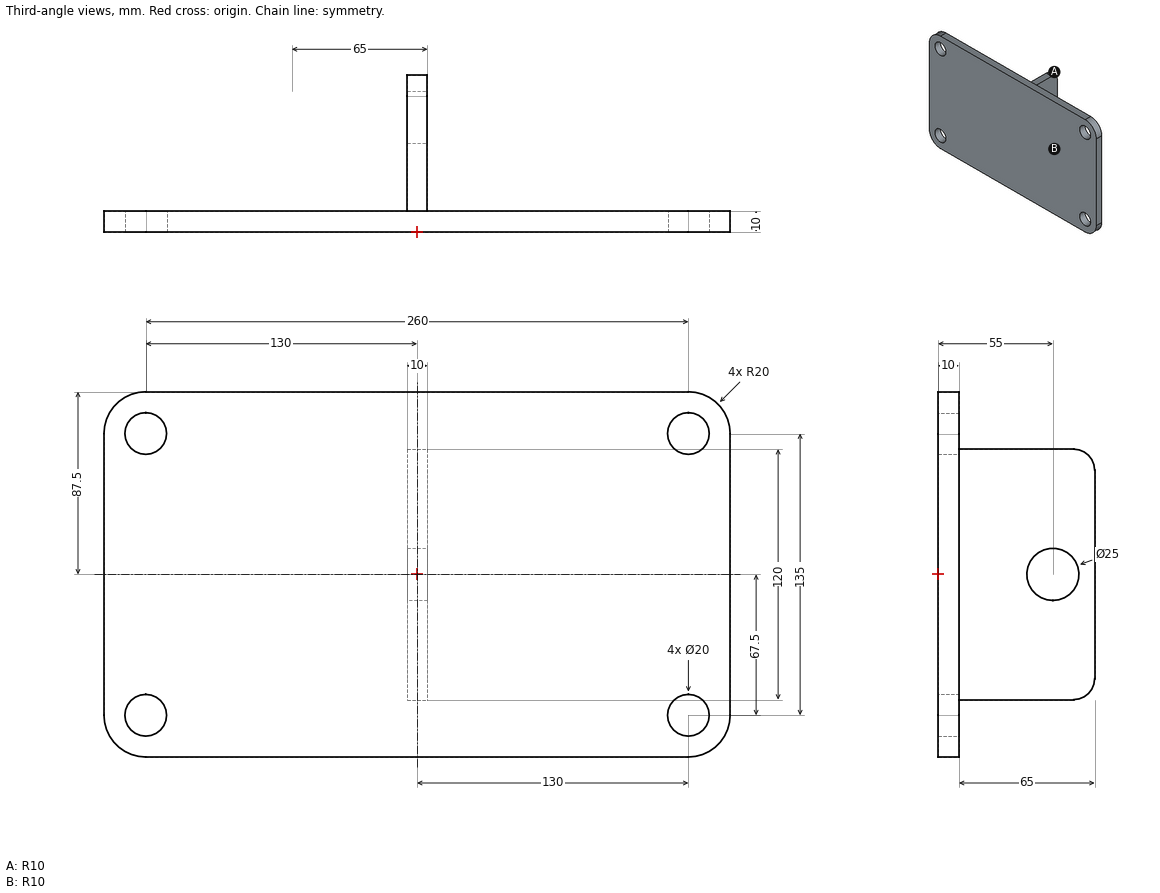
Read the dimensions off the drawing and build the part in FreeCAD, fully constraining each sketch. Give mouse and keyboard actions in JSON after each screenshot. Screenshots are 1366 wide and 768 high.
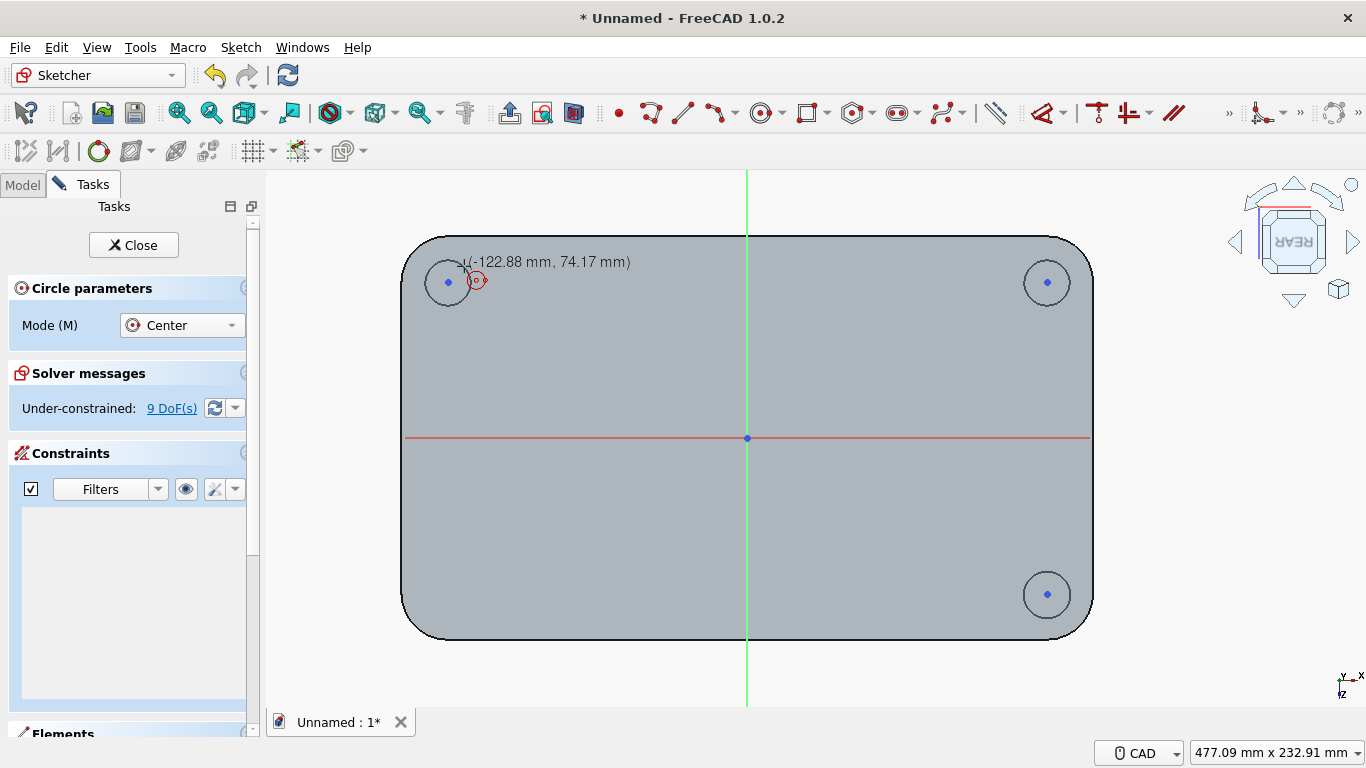
{"action": "left_click", "coordinate": [448, 594]}
{"action": "left_click", "coordinate": [464, 577]}
{"action": "key", "text": "Escape"}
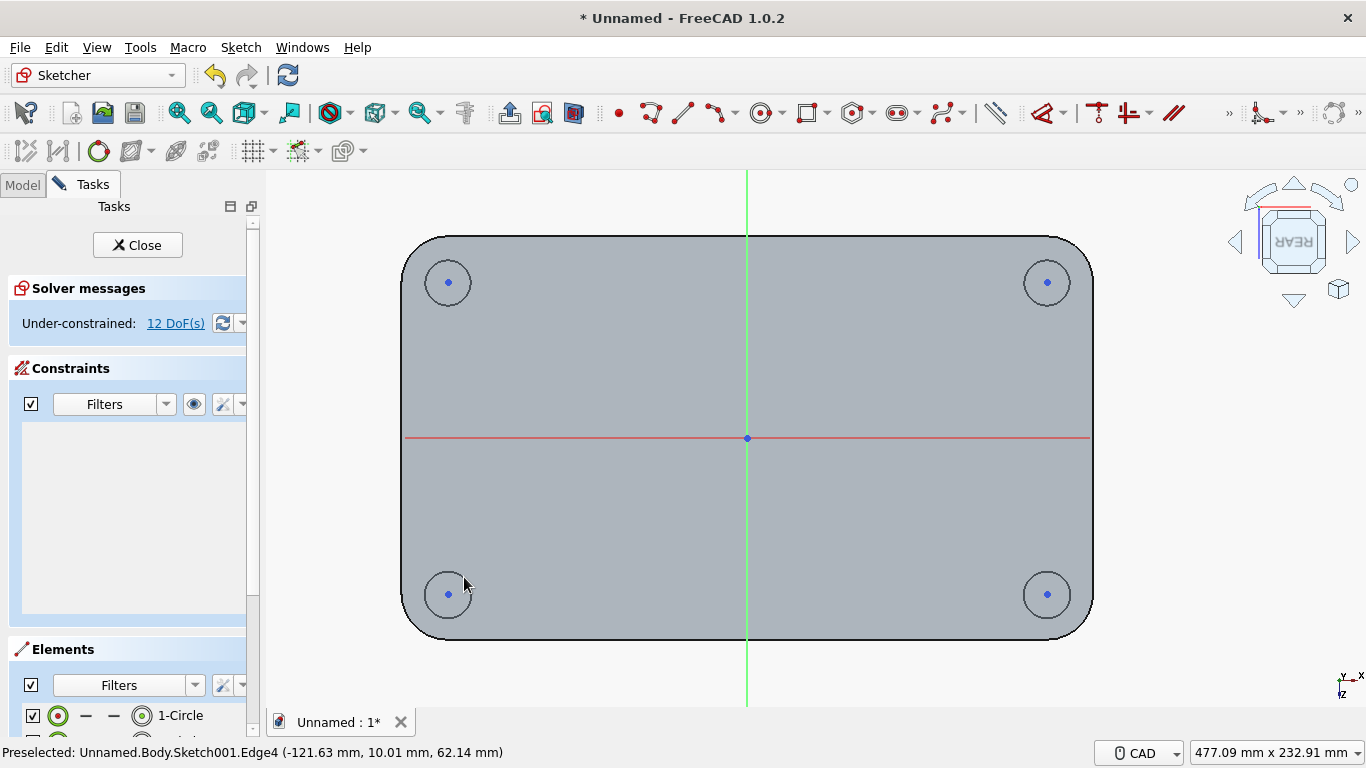
{"action": "left_click", "coordinate": [1063, 267]}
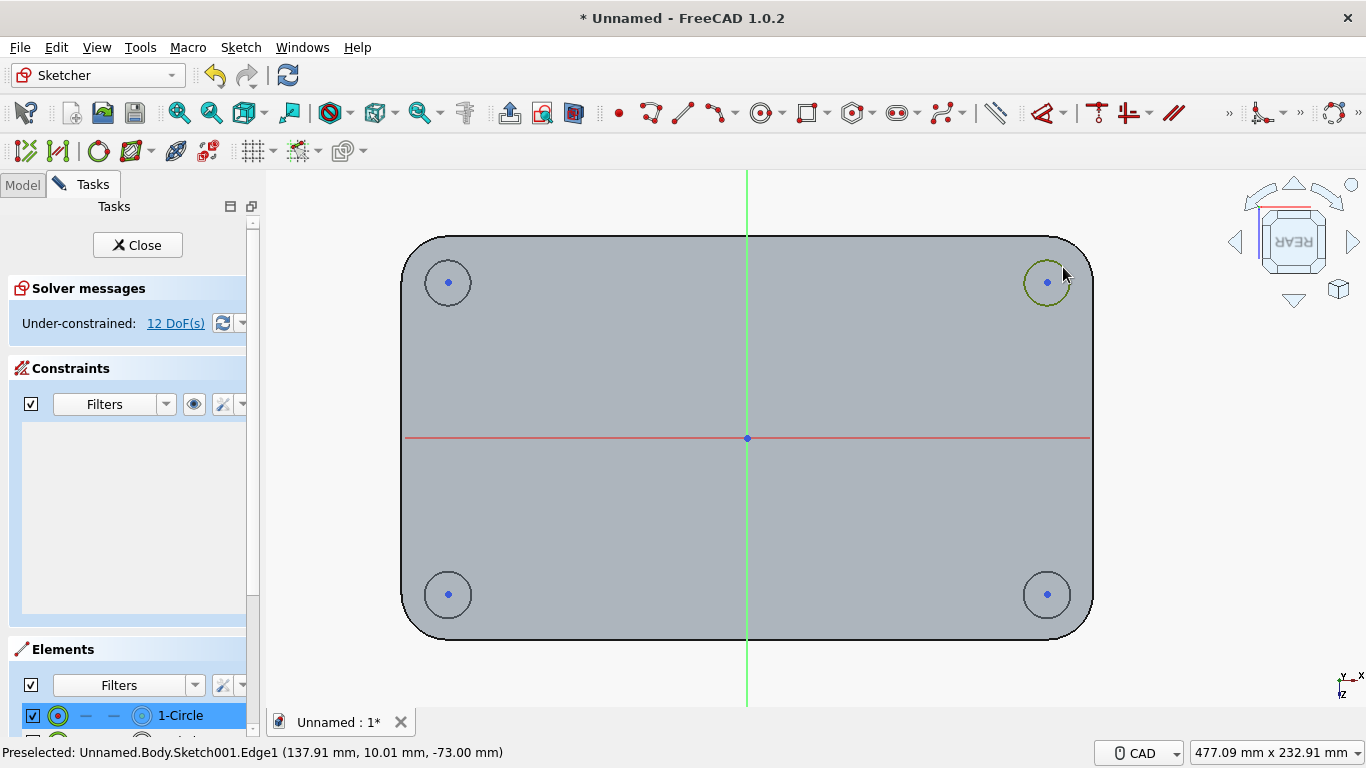
{"action": "left_click", "coordinate": [1063, 578]}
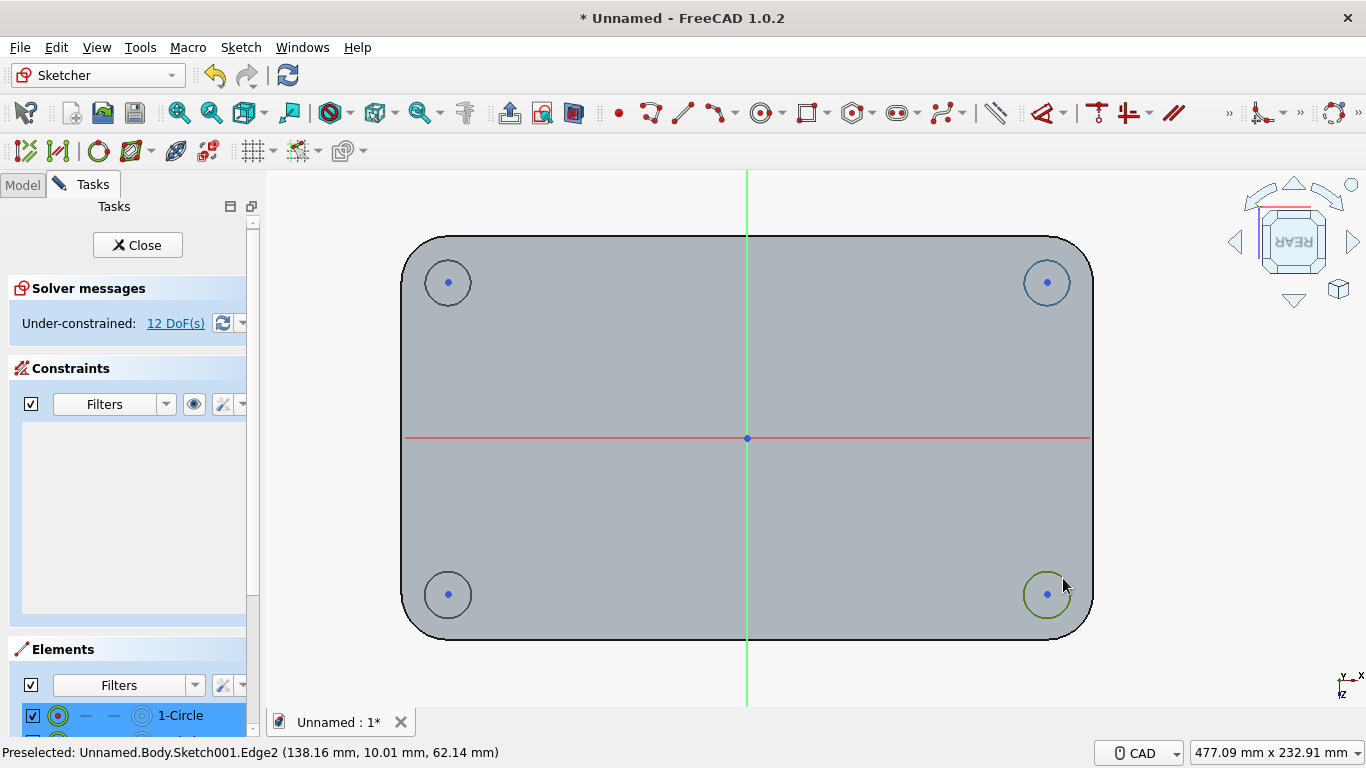
{"action": "left_click", "coordinate": [464, 267]}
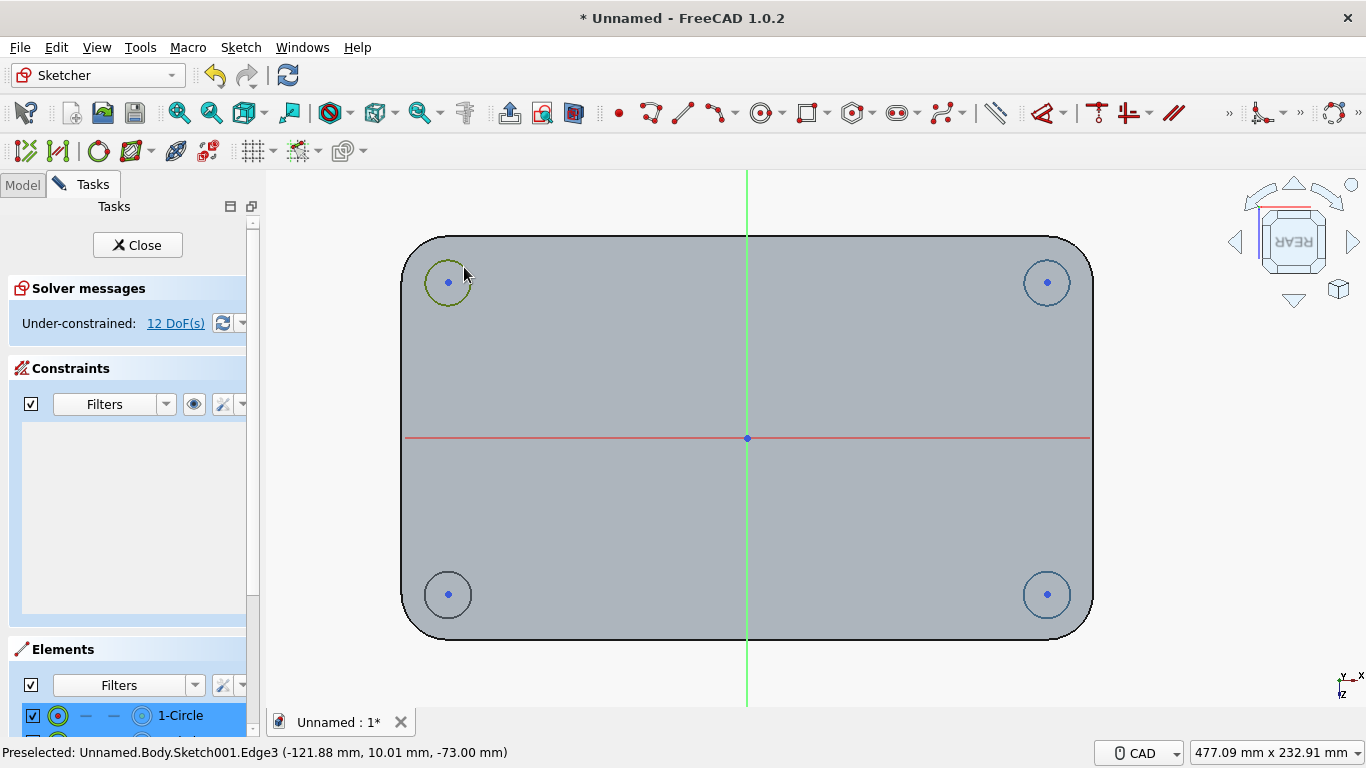
{"action": "left_click", "coordinate": [464, 578]}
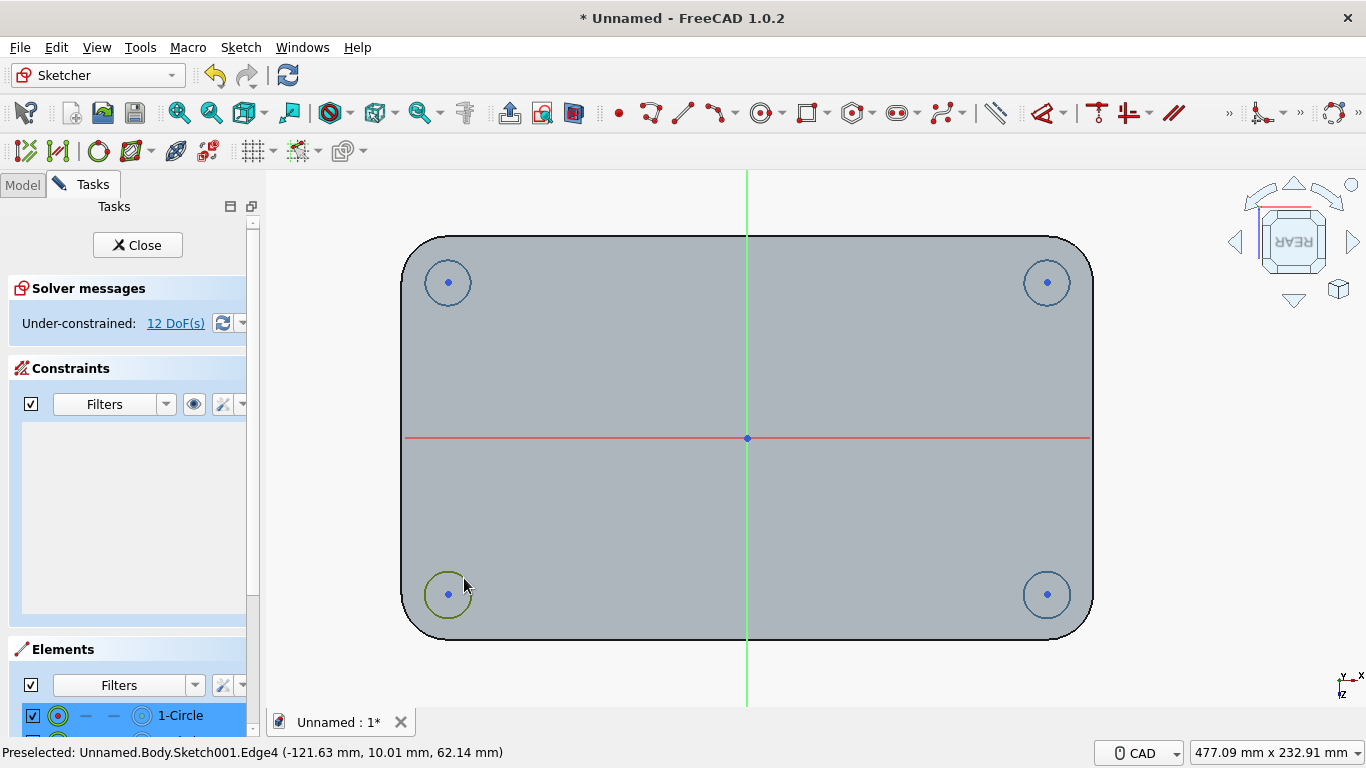
{"action": "key", "text": "e"}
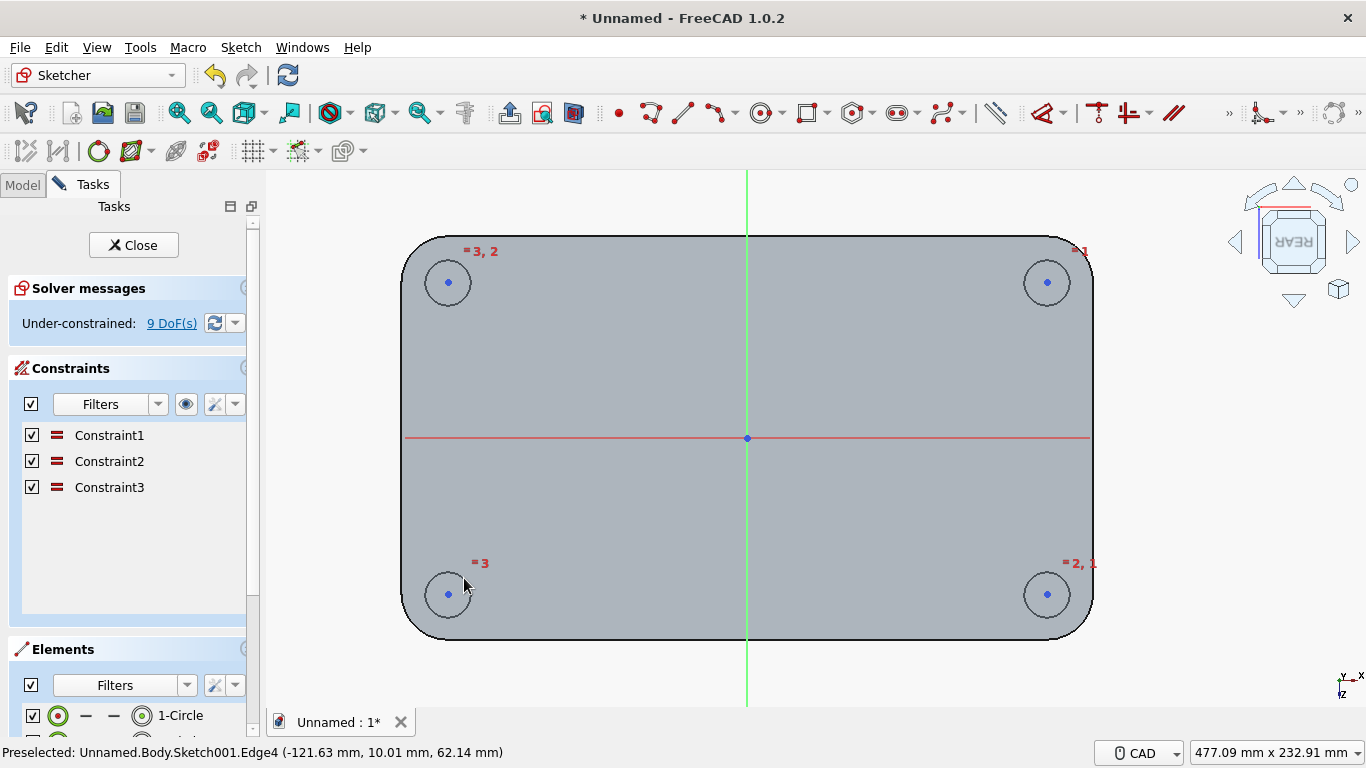
{"action": "left_click", "coordinate": [1047, 283]}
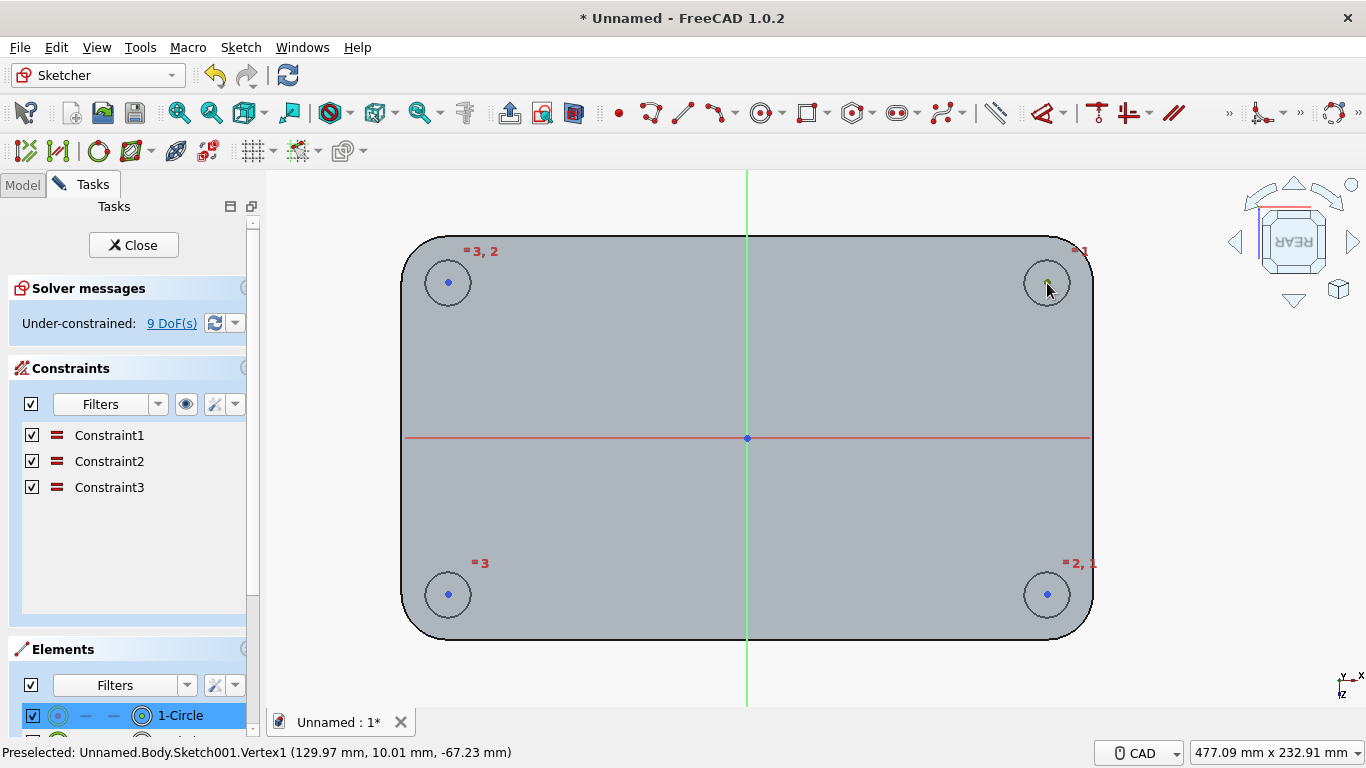
{"action": "left_click", "coordinate": [1047, 595]}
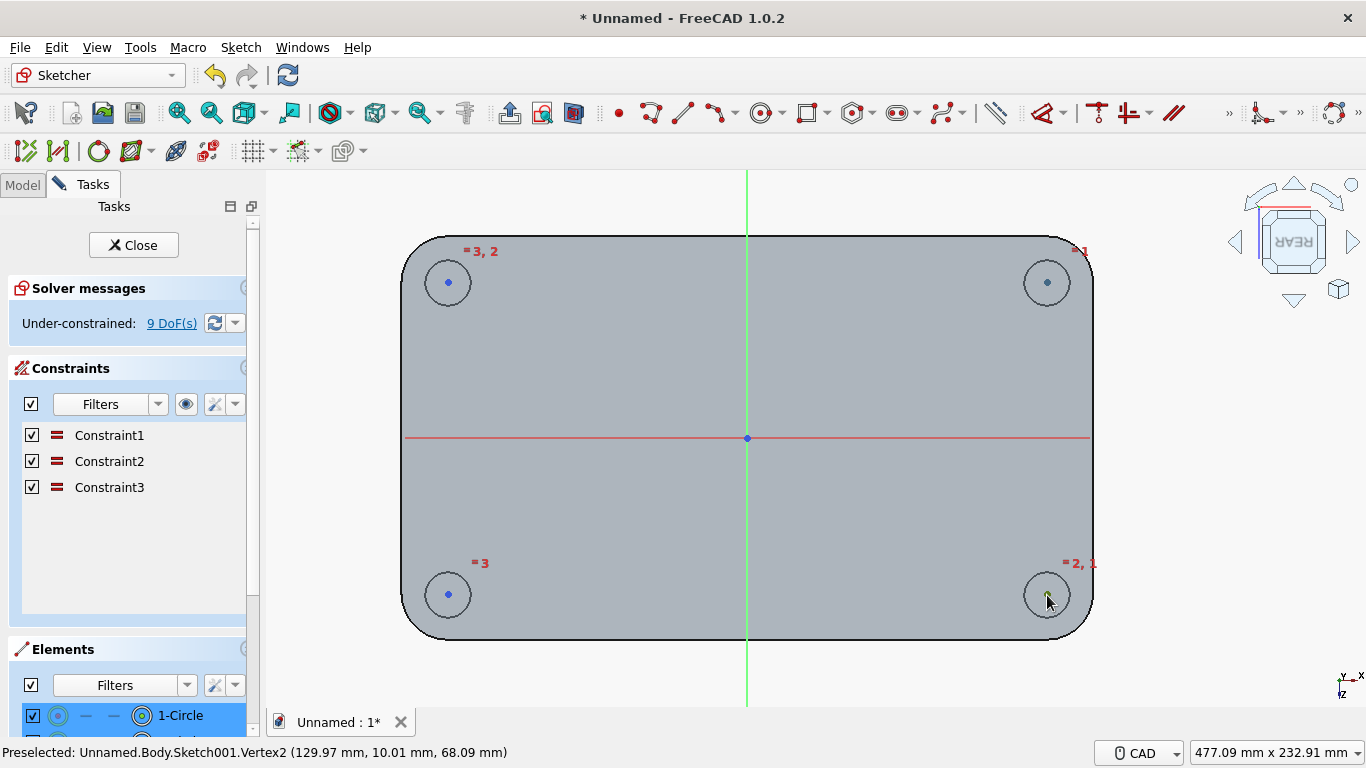
{"action": "left_click", "coordinate": [424, 438]}